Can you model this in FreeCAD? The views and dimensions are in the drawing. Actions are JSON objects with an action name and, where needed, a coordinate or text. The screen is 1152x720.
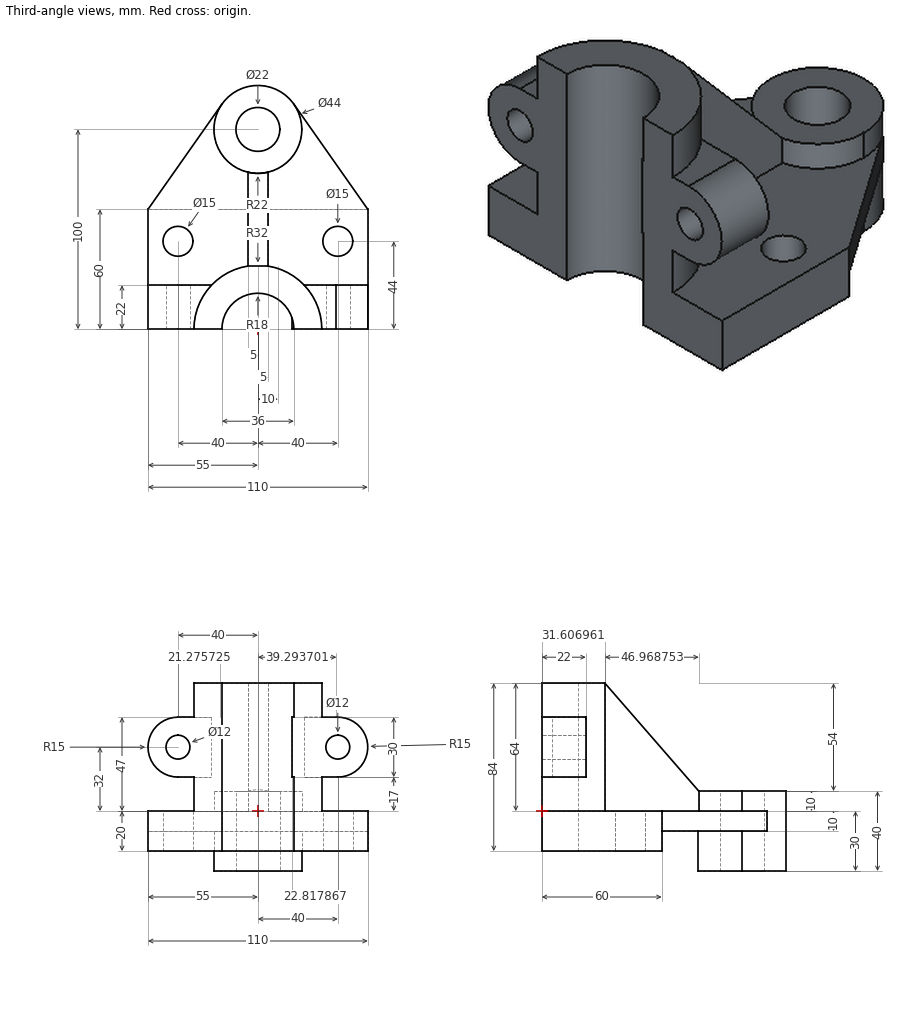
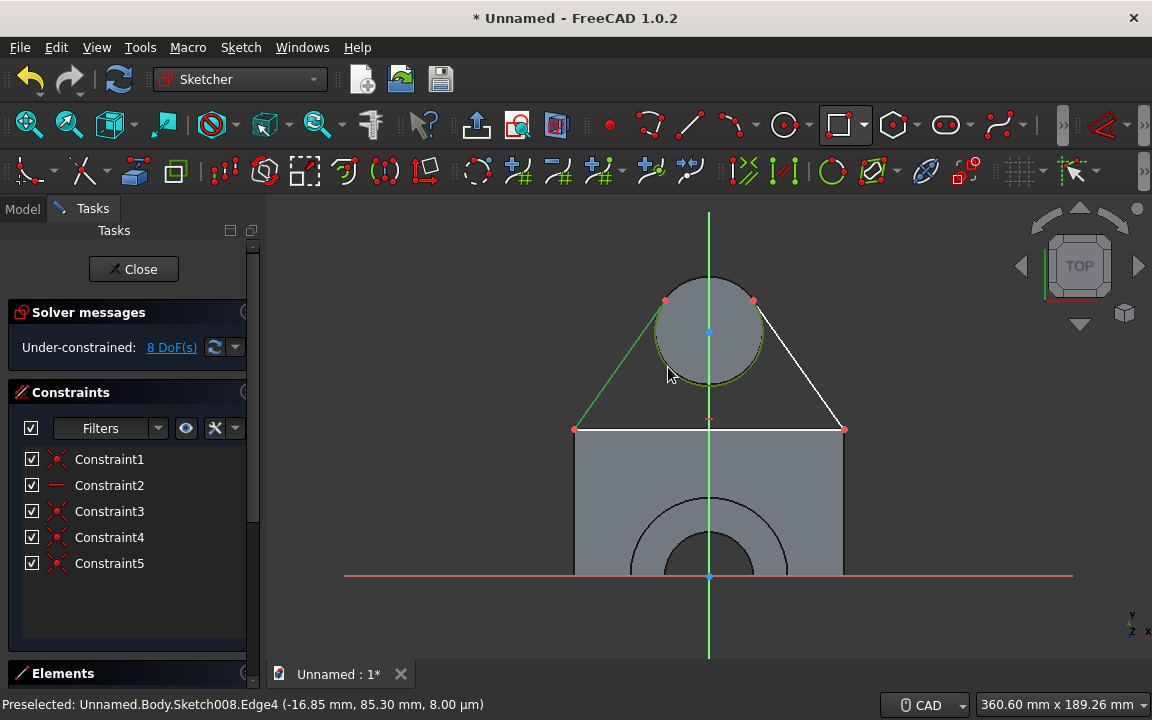
{"action": "key", "text": "t"}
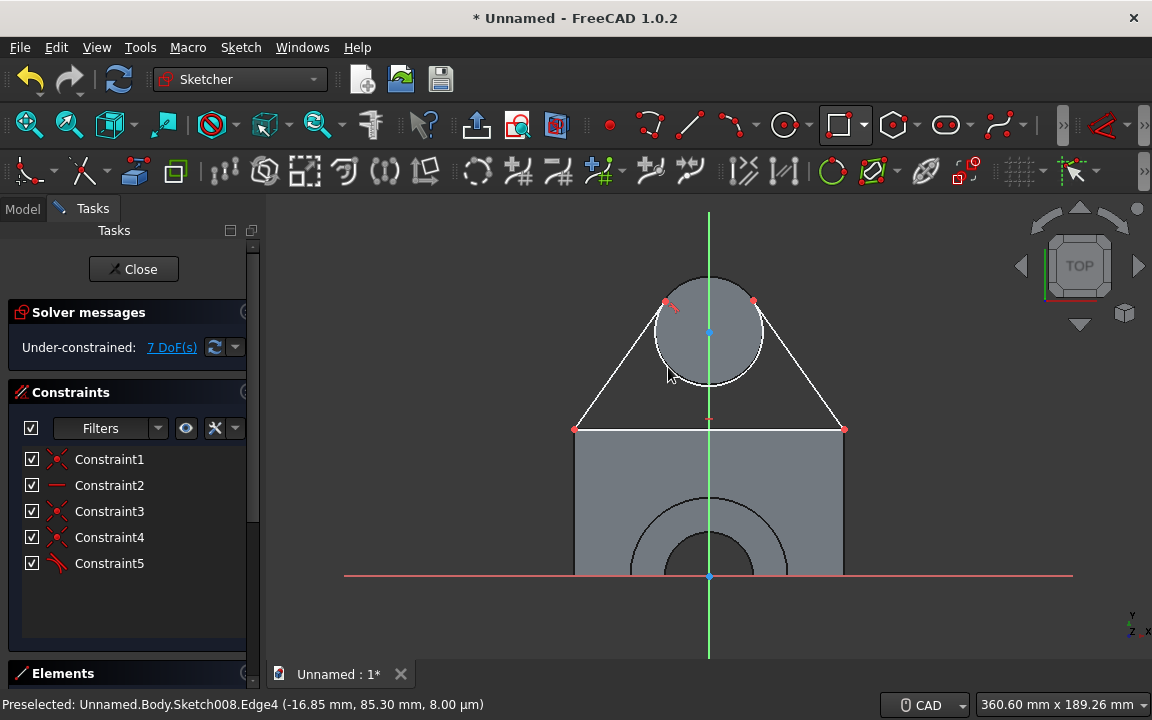
{"action": "left_click", "coordinate": [817, 391]}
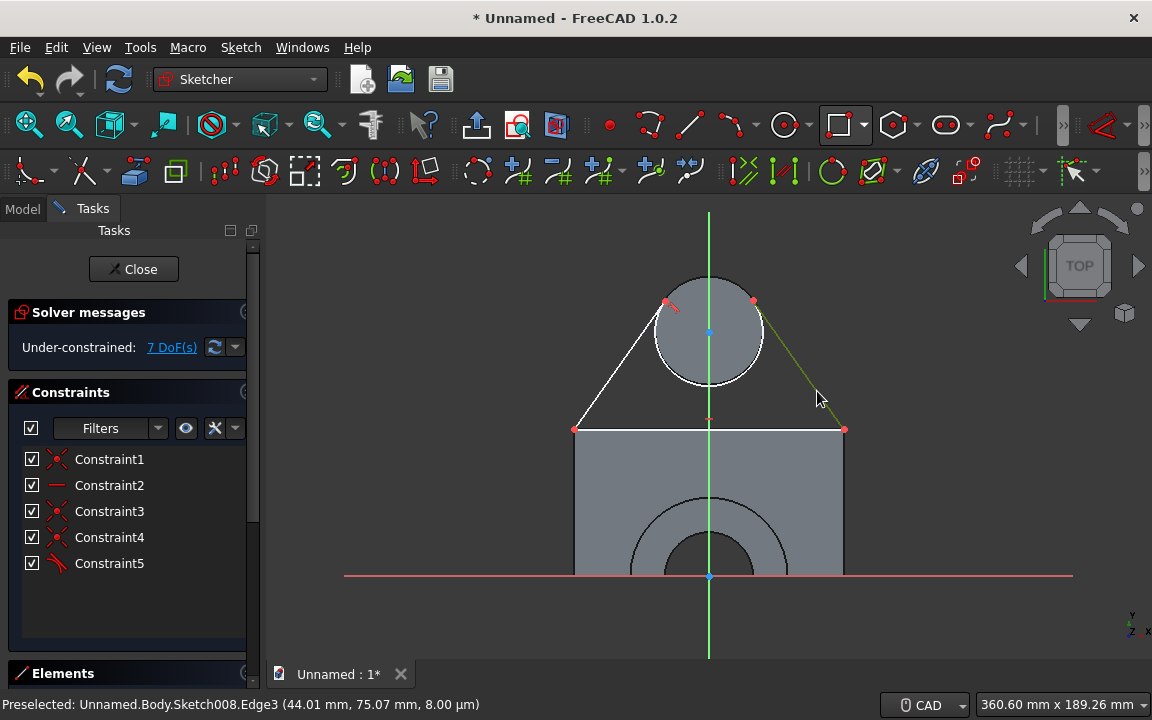
{"action": "left_click", "coordinate": [668, 367]}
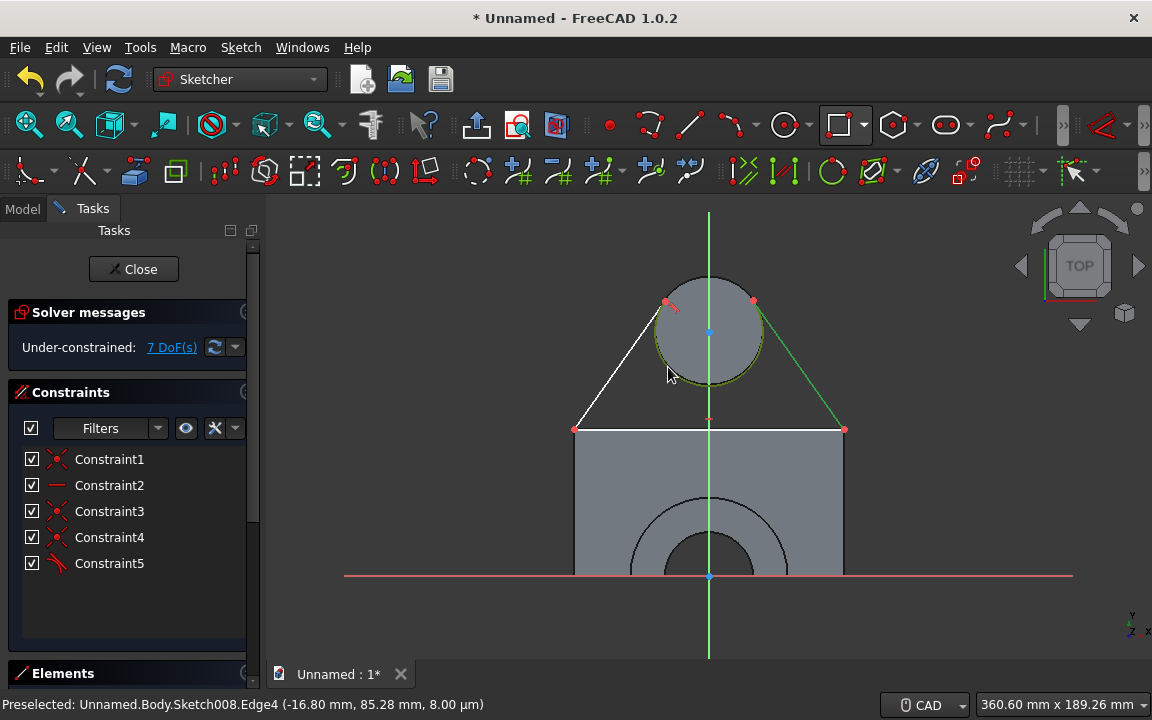
{"action": "key", "text": "t"}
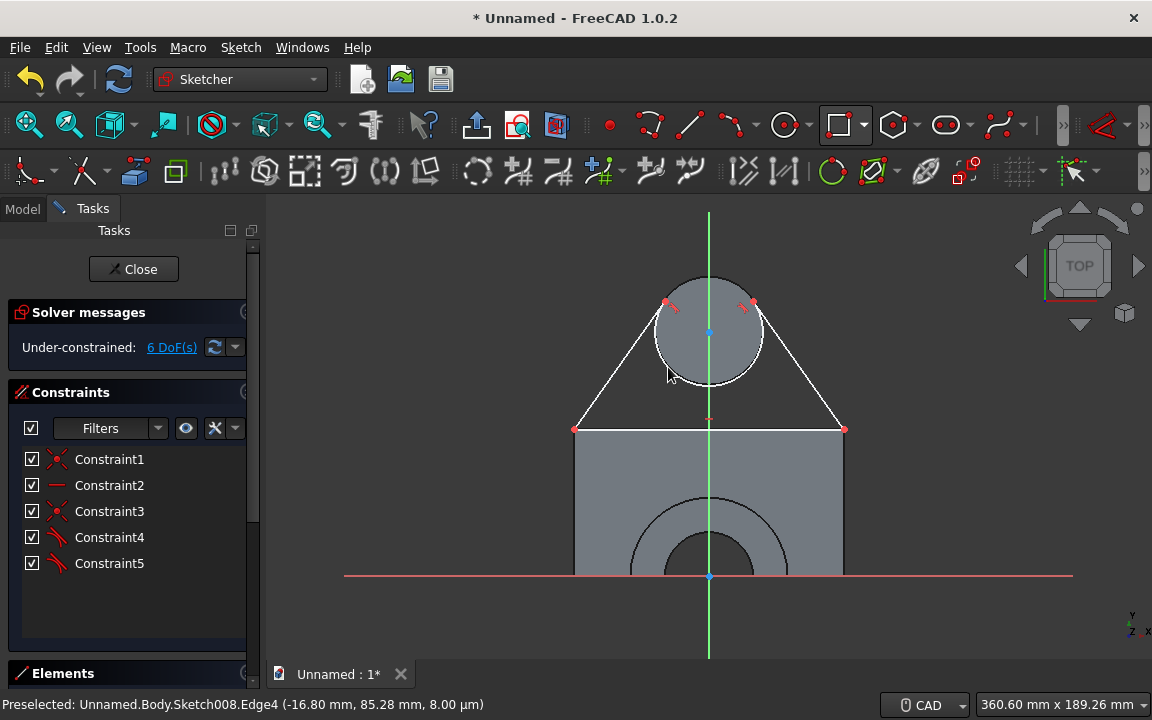
{"action": "left_click", "coordinate": [709, 332]}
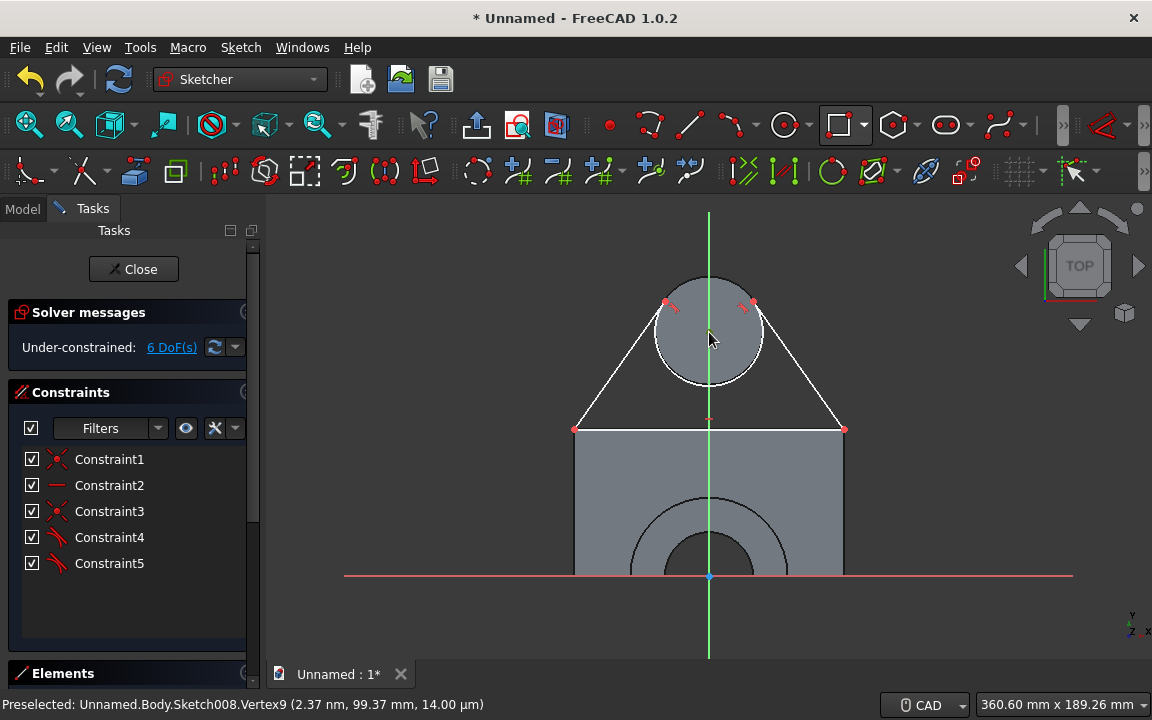
{"action": "left_click", "coordinate": [709, 543]}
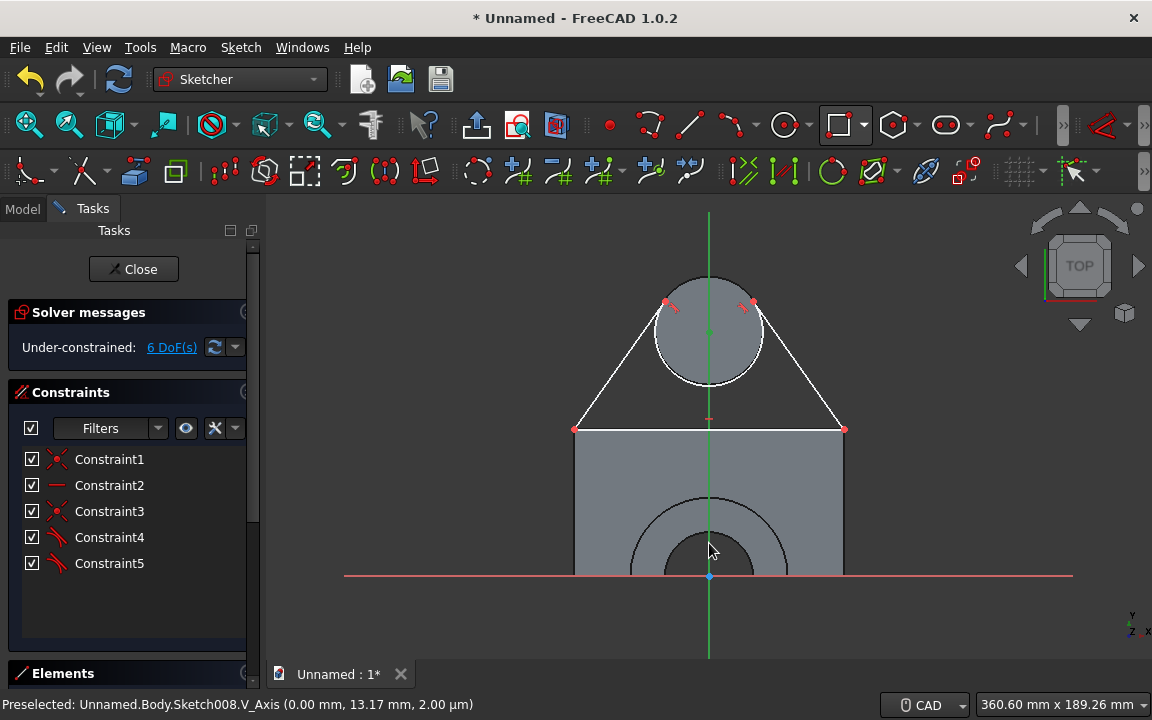
{"action": "key", "text": "c"}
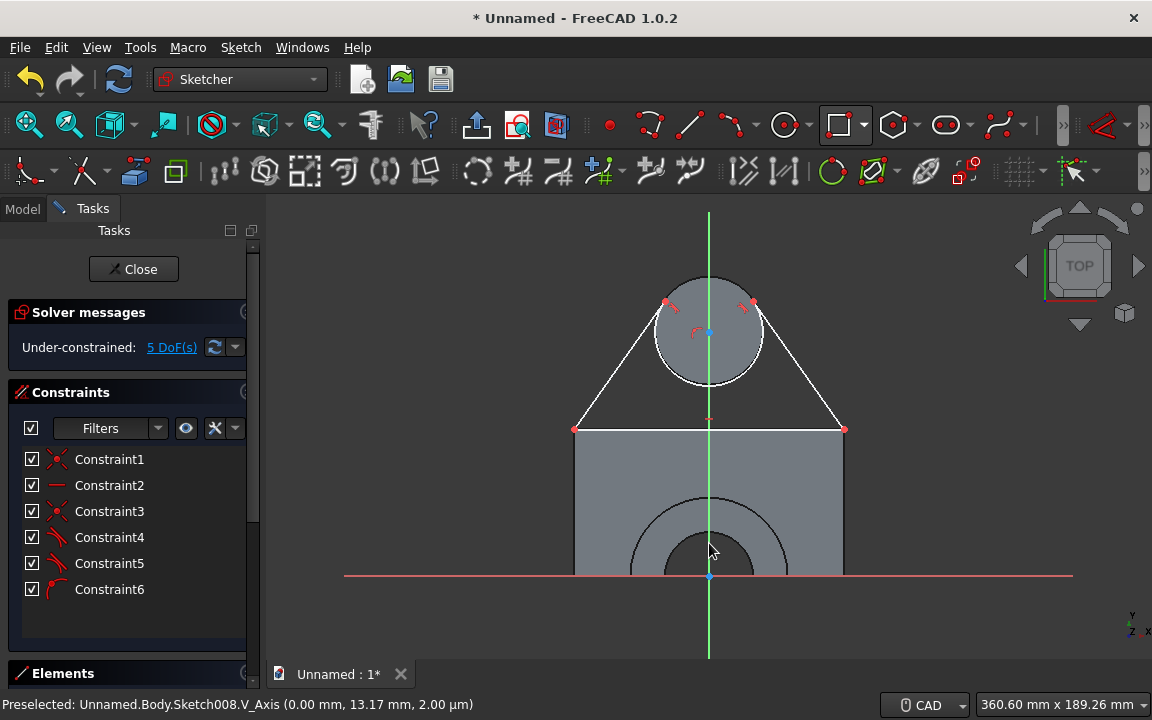
{"action": "left_click", "coordinate": [1102, 126]}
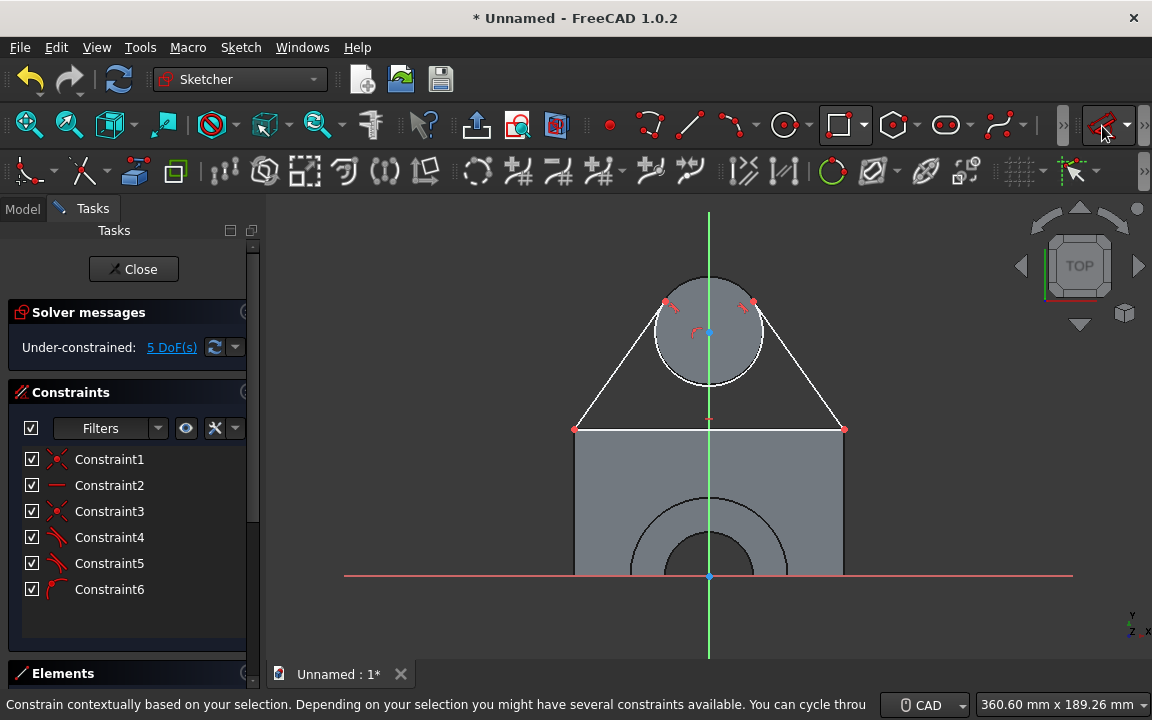
{"action": "left_click", "coordinate": [668, 367]}
{"action": "left_click", "coordinate": [644, 388]}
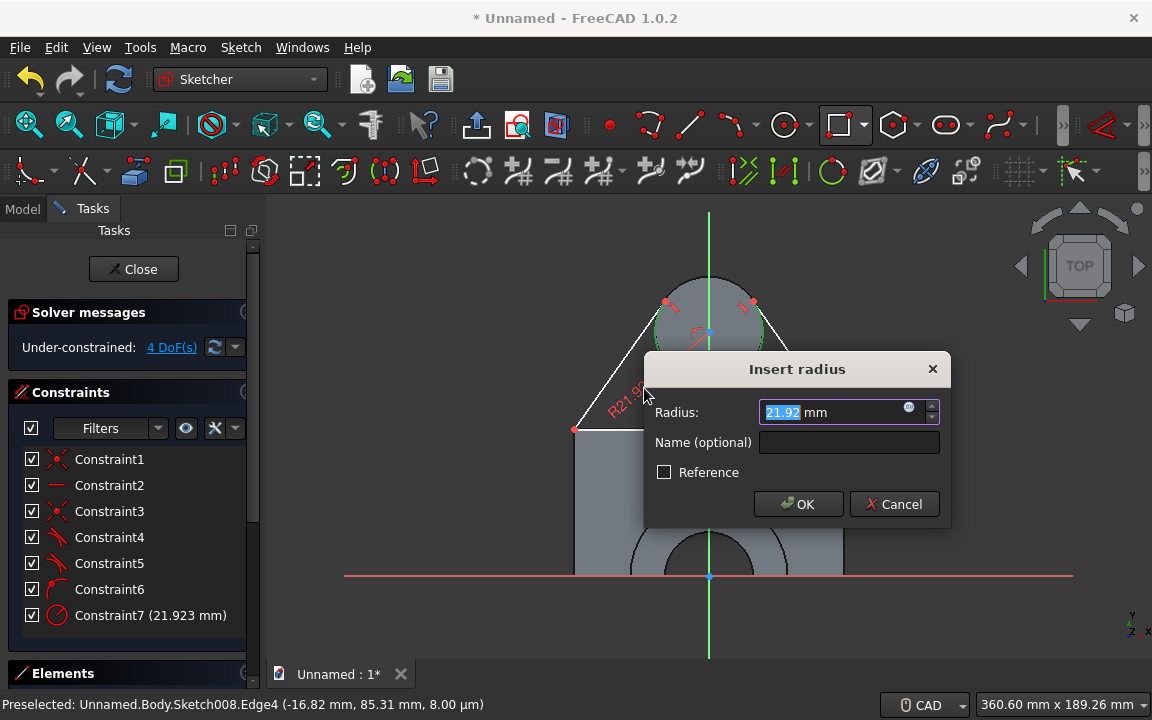
{"action": "type", "text": "22"}
{"action": "key", "text": "Return"}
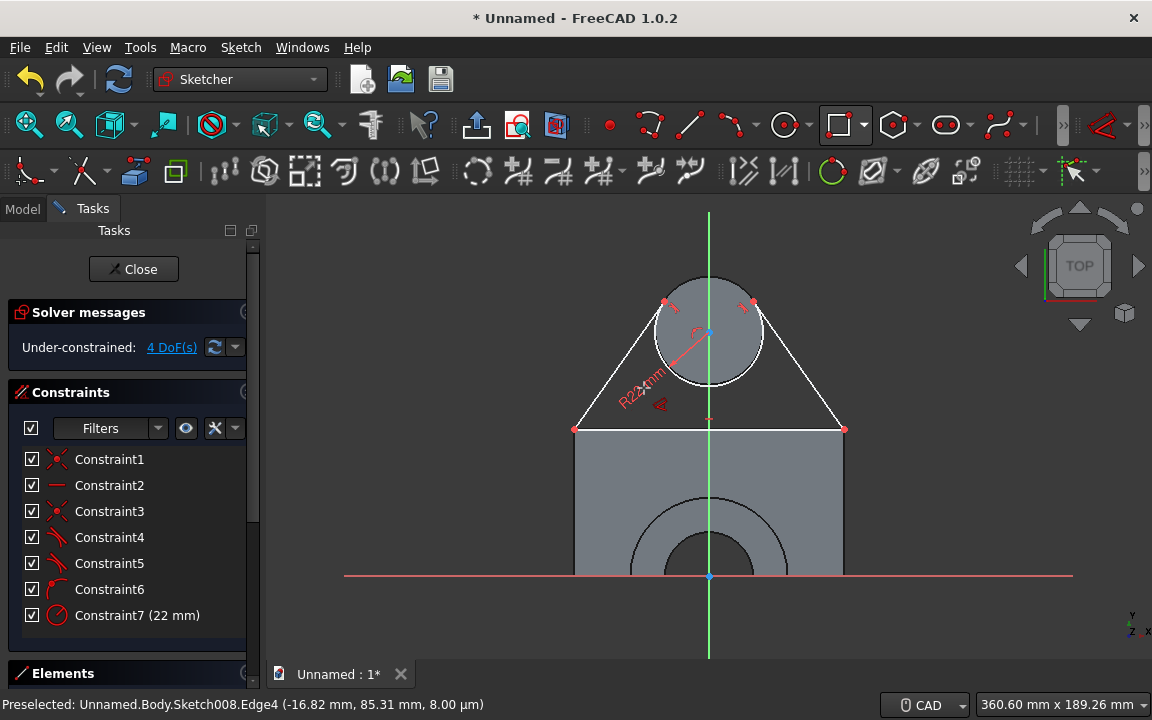
{"action": "left_click", "coordinate": [655, 430]}
{"action": "left_click", "coordinate": [771, 396]}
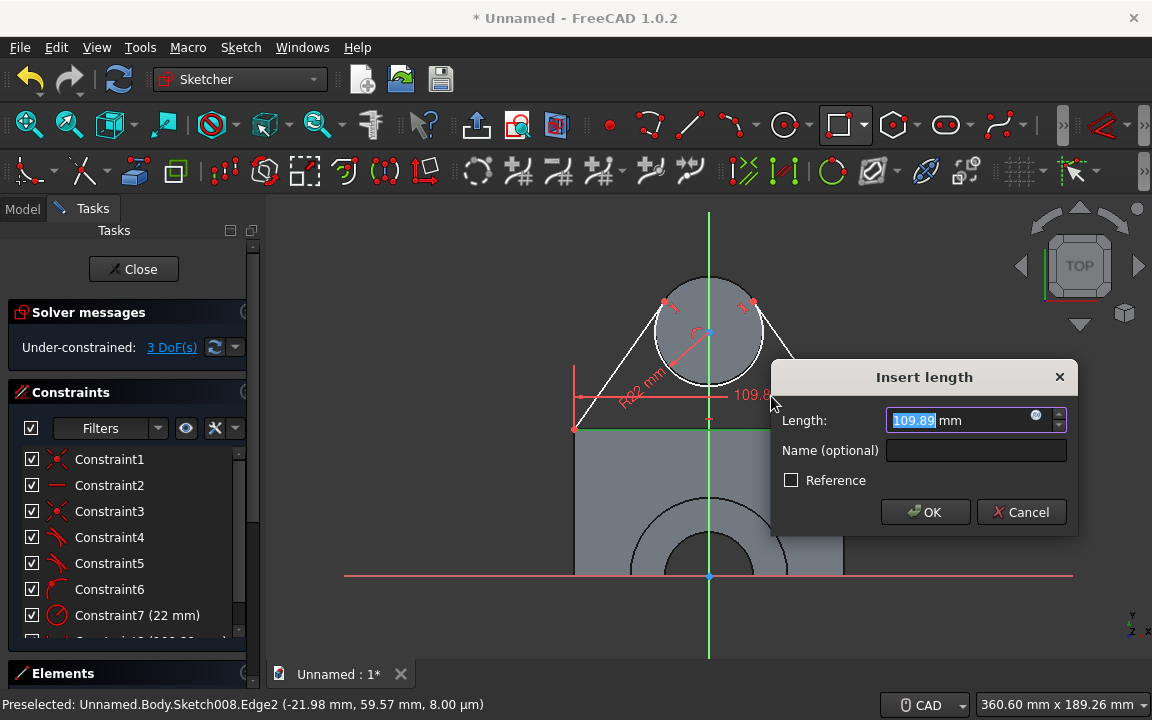
{"action": "type", "text": "110"}
{"action": "key", "text": "Return"}